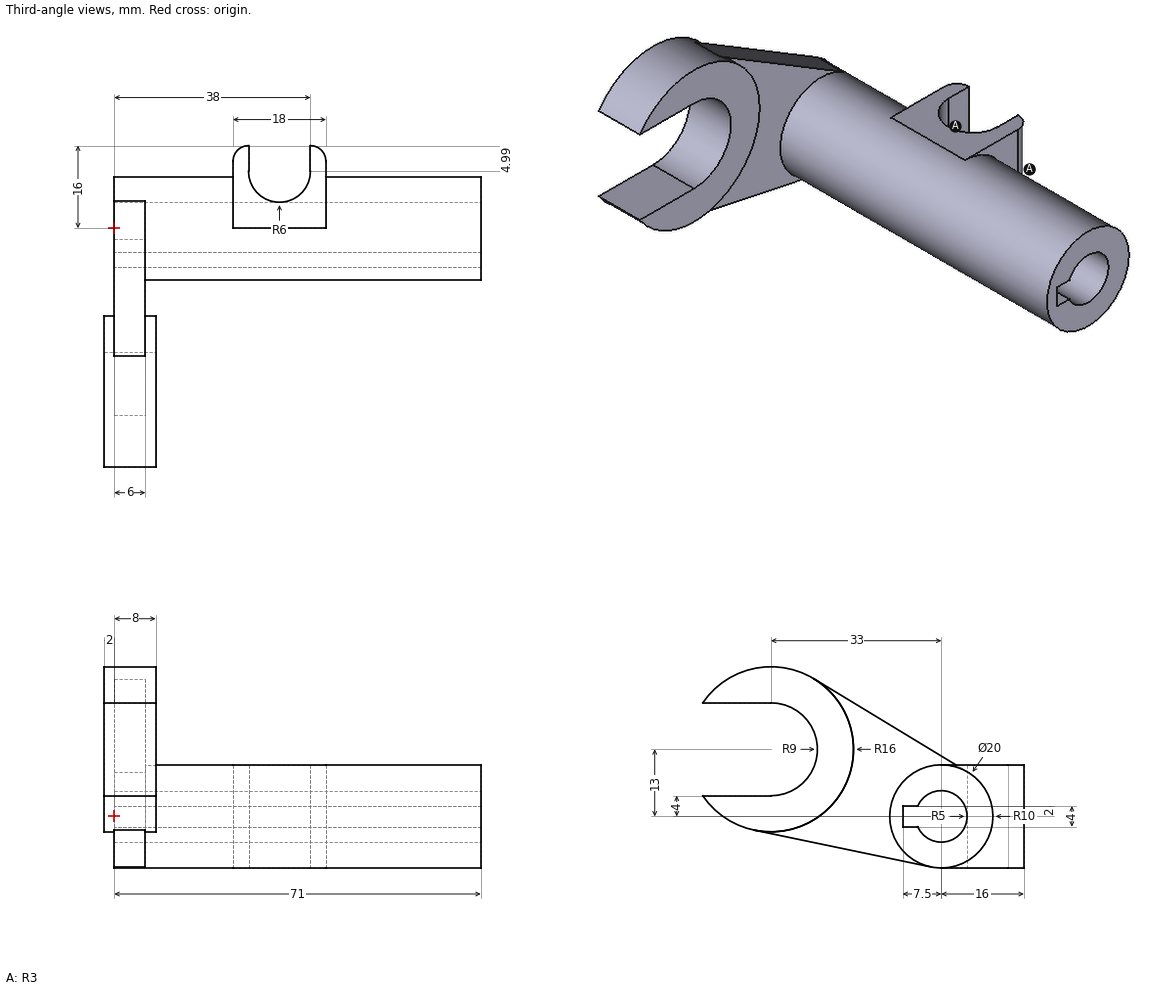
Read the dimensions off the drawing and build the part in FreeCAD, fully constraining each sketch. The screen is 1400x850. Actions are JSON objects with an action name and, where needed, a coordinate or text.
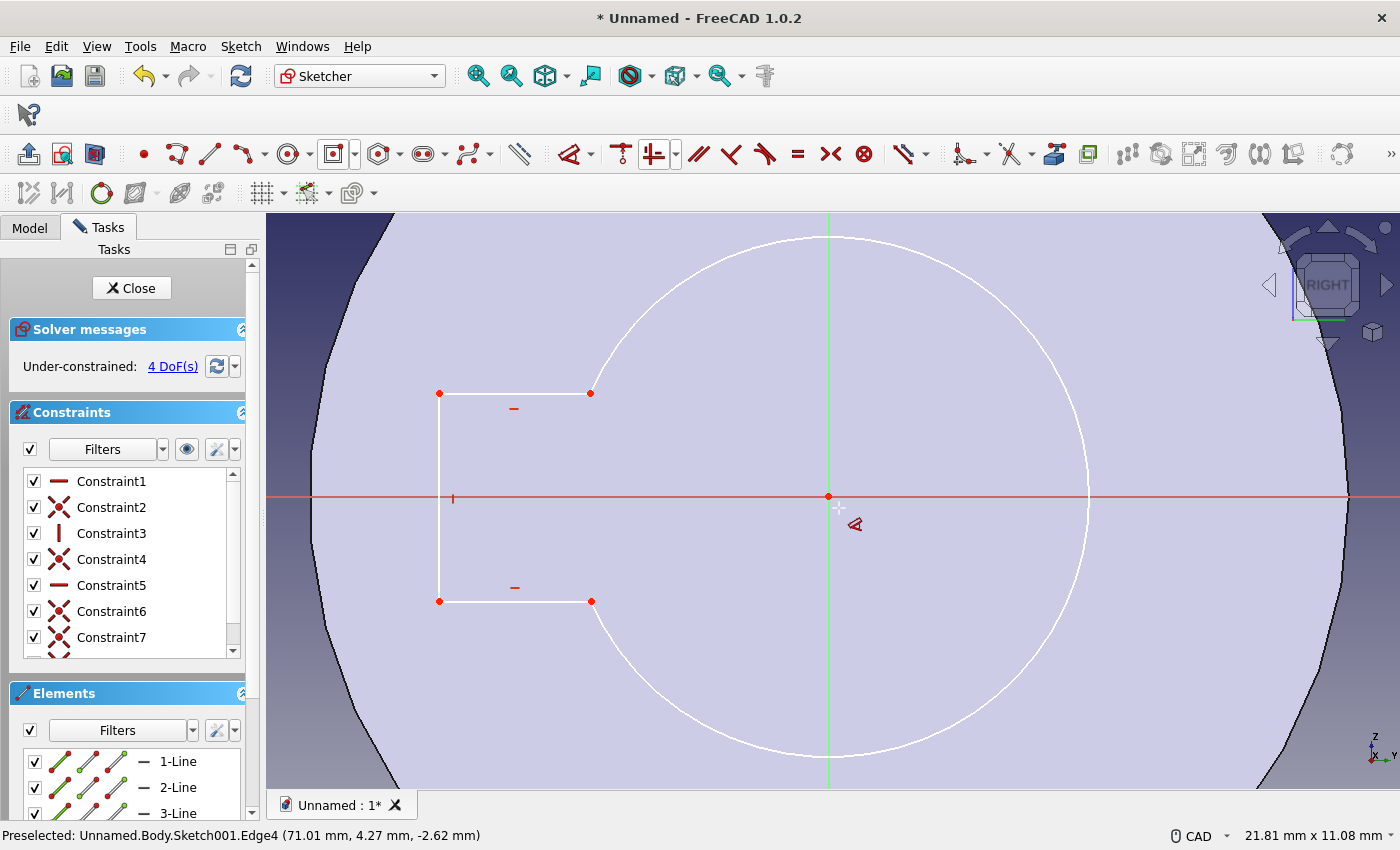
{"action": "left_click", "coordinate": [950, 727]}
{"action": "left_click", "coordinate": [965, 755]}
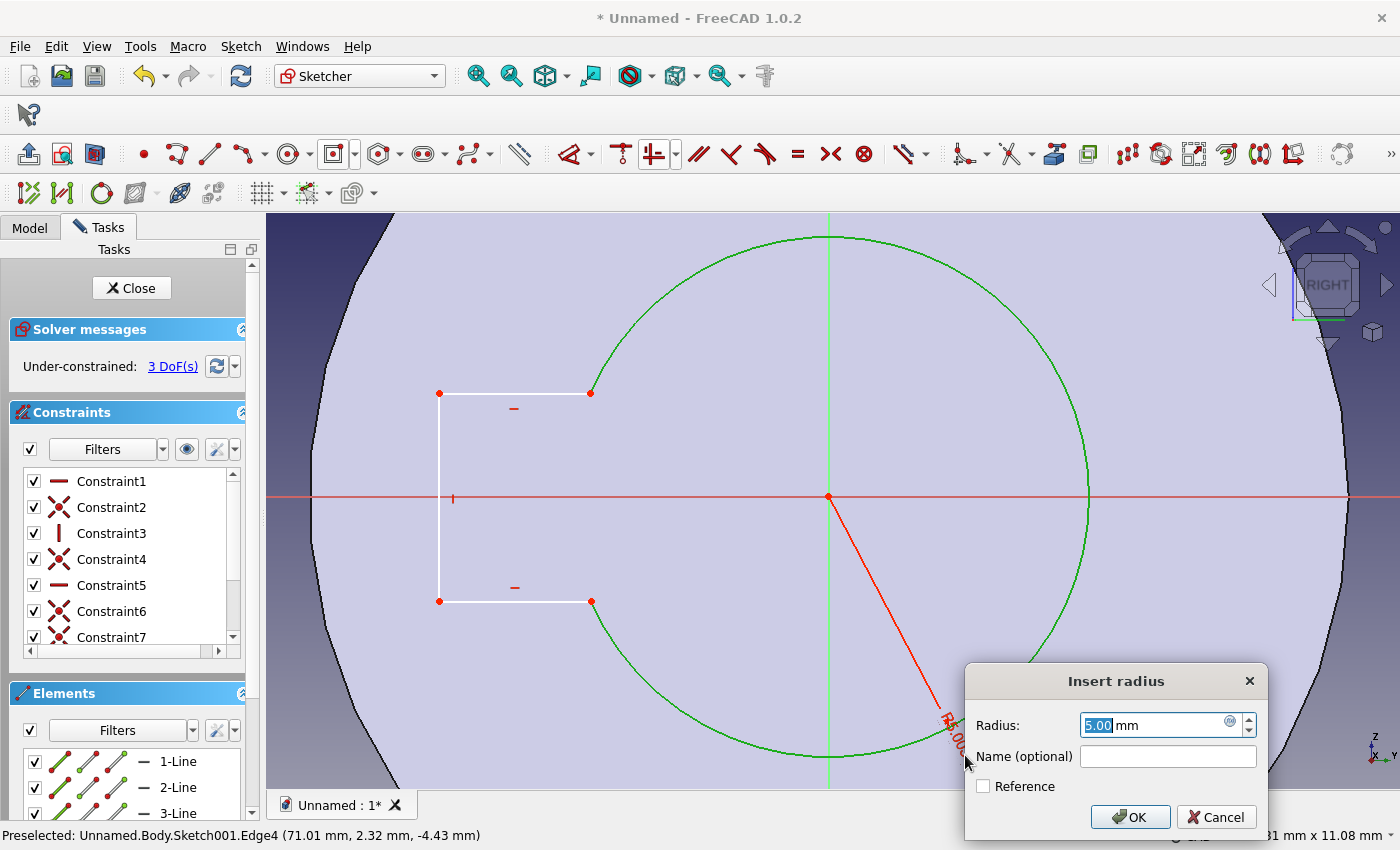
{"action": "type", "text": "5"}
{"action": "key", "text": "Return"}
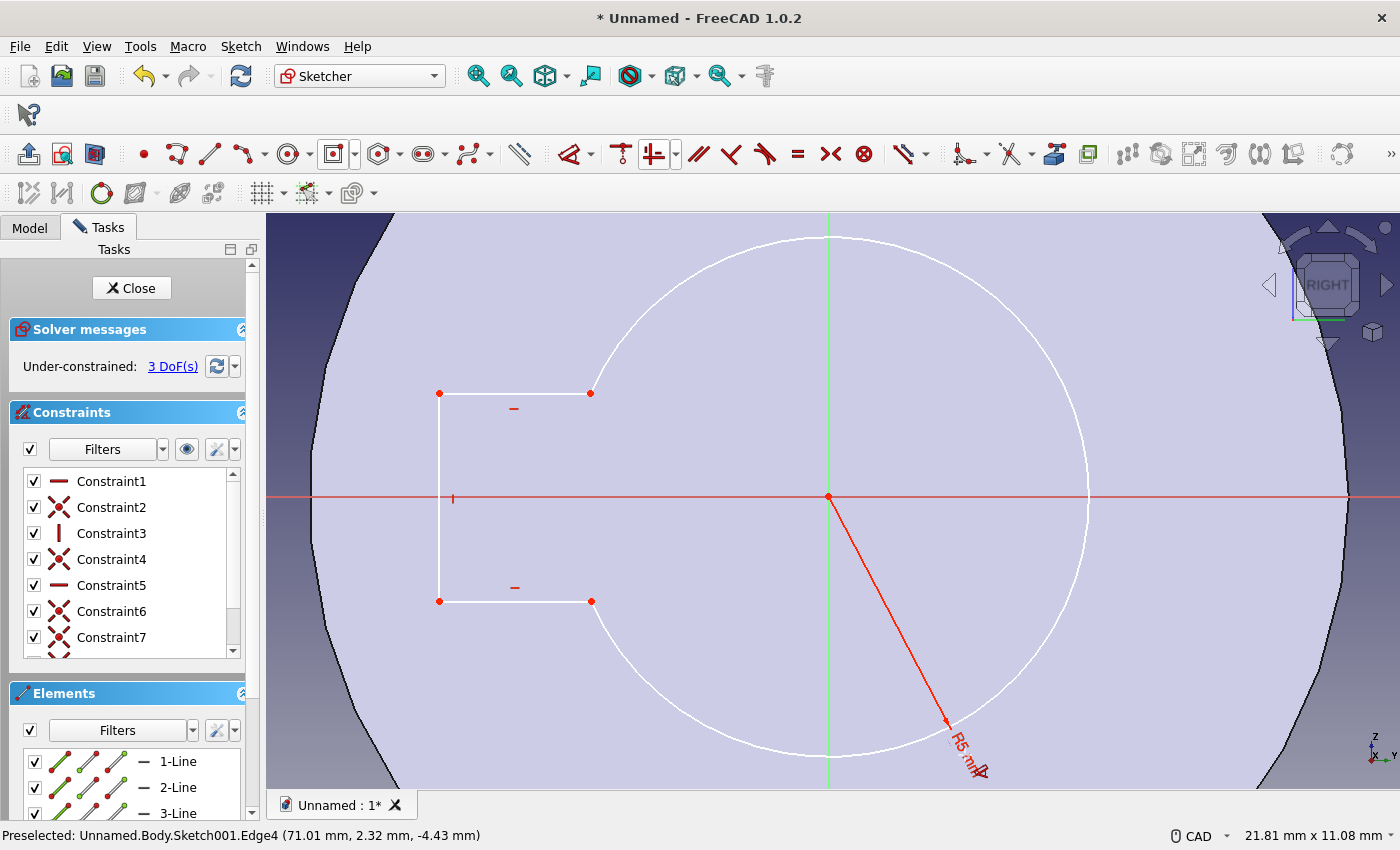
{"action": "left_click", "coordinate": [439, 456]}
{"action": "left_click", "coordinate": [405, 450]}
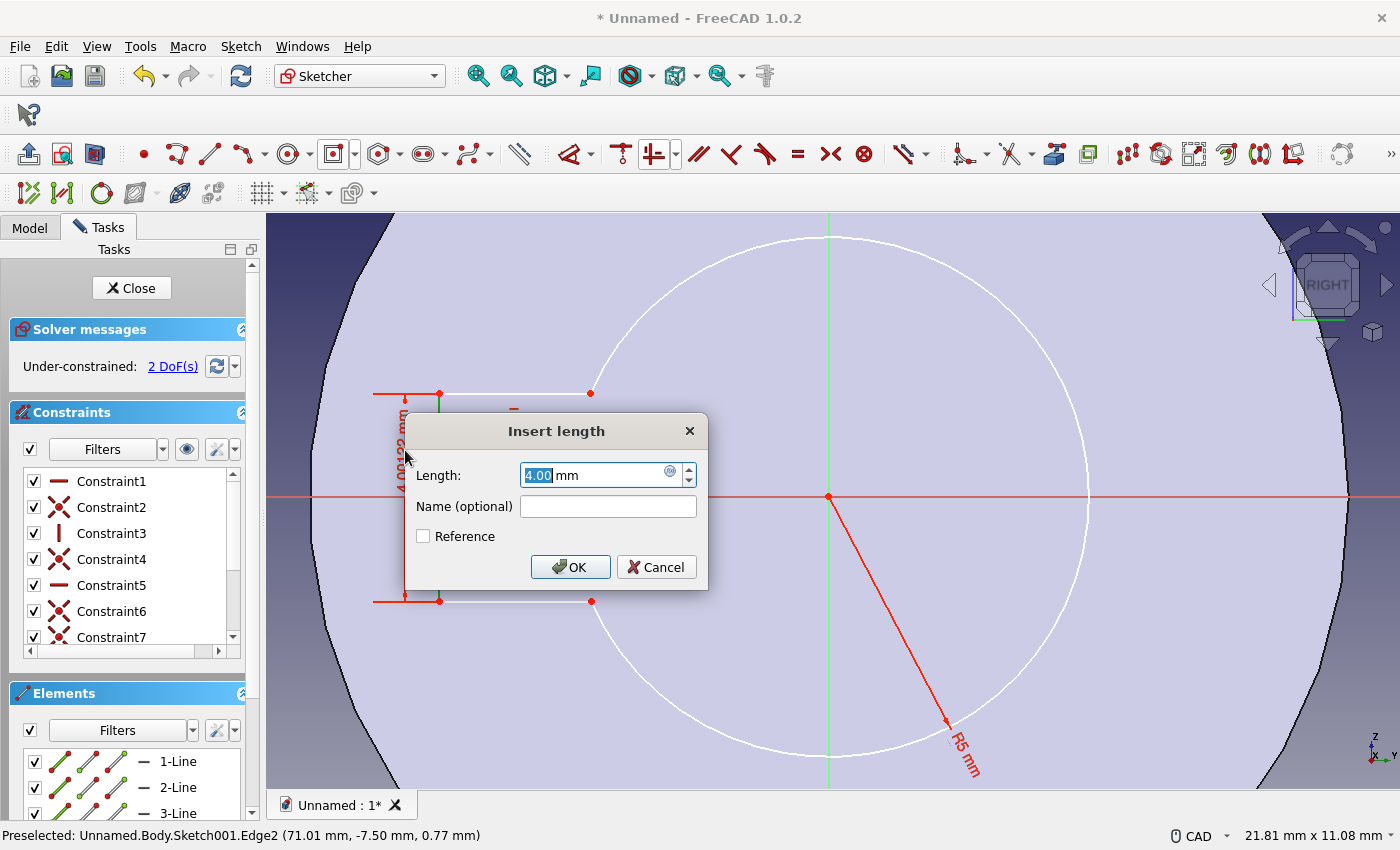
{"action": "type", "text": "4"}
{"action": "key", "text": "Return"}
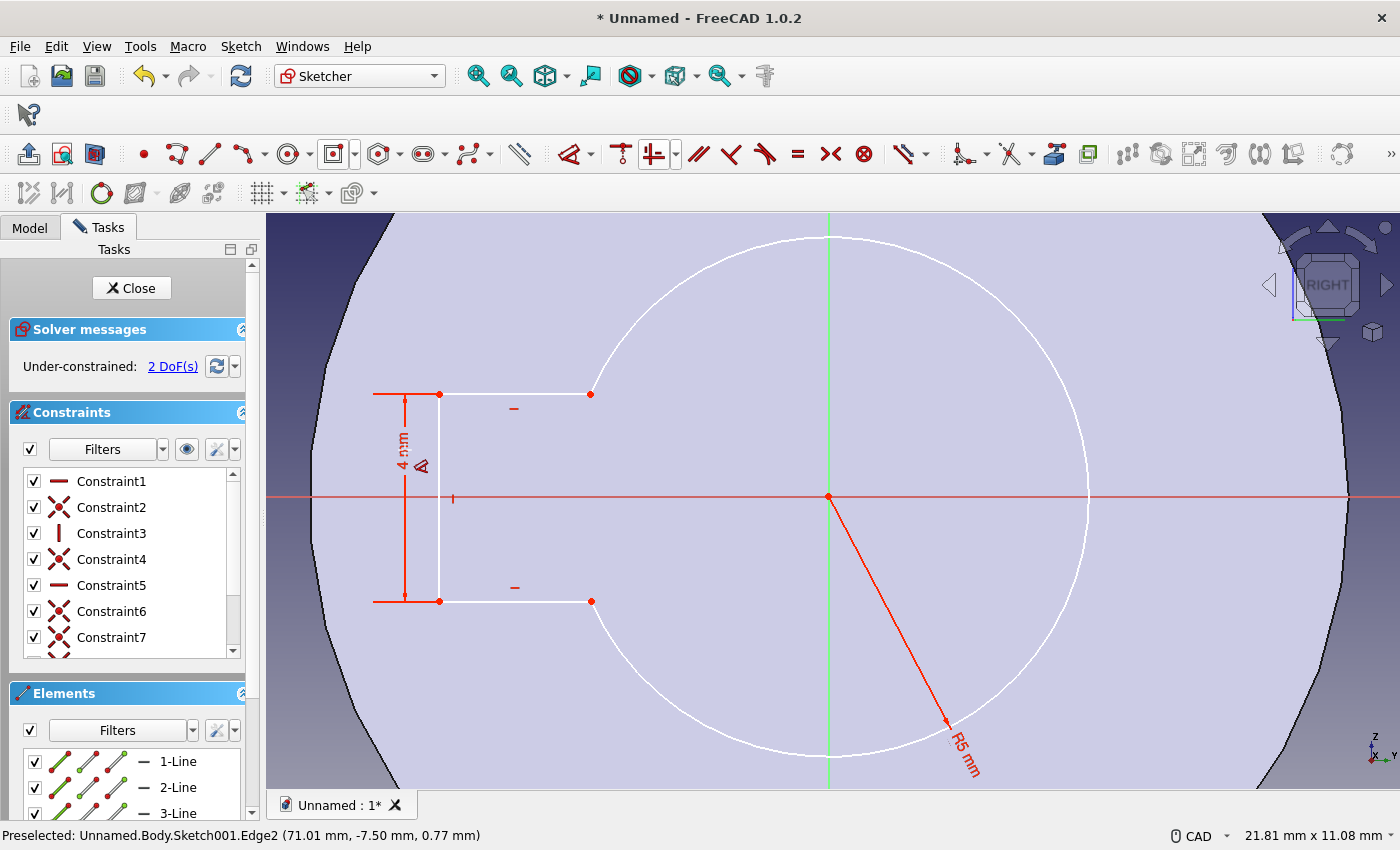
{"action": "left_click", "coordinate": [590, 394]}
{"action": "left_click", "coordinate": [556, 446]}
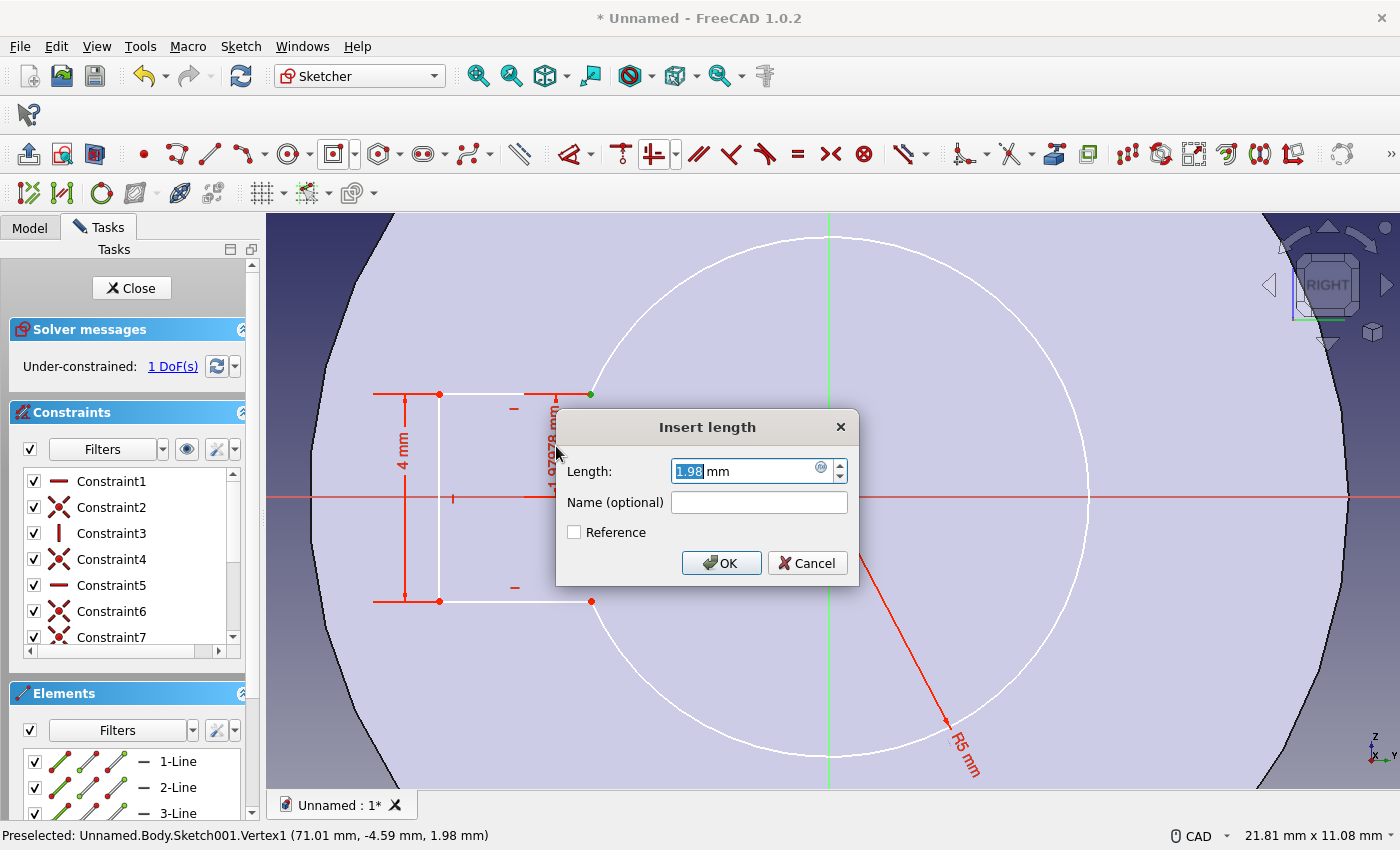
{"action": "type", "text": "2"}
{"action": "key", "text": "Return"}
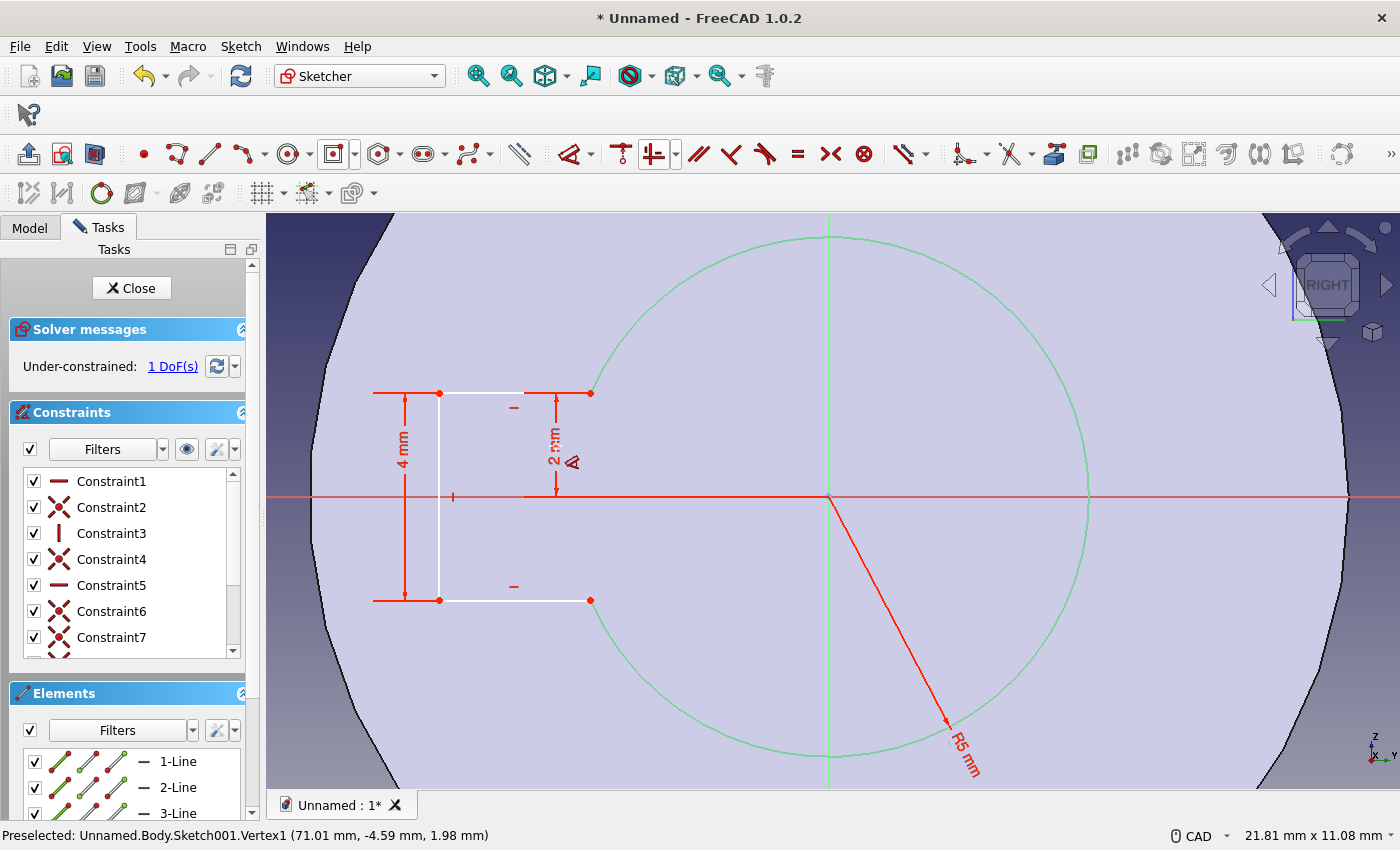
{"action": "left_click", "coordinate": [439, 393]}
{"action": "left_click", "coordinate": [634, 359]}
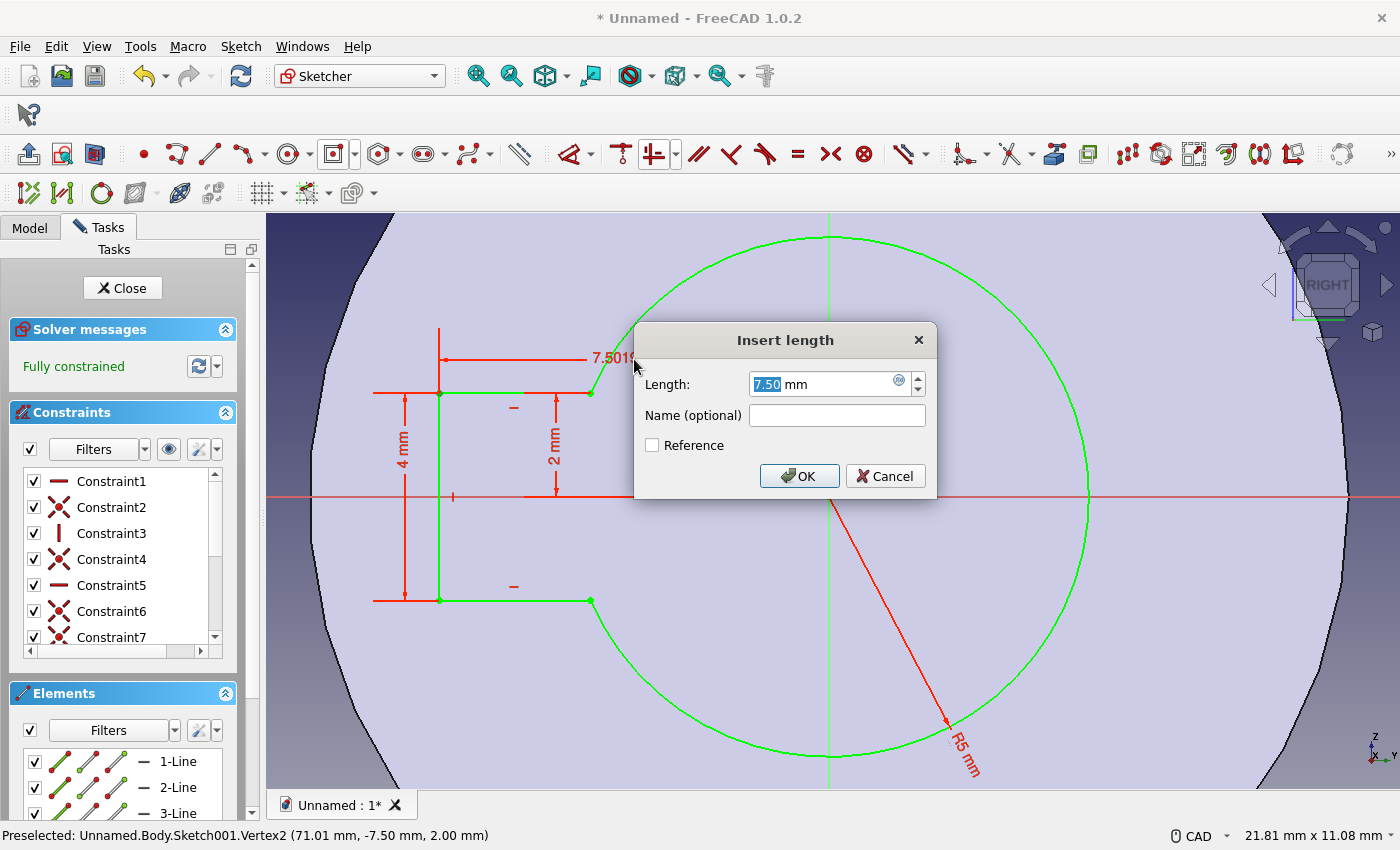
{"action": "type", "text": "7.5"}
{"action": "key", "text": "Return"}
{"action": "key", "text": "Escape"}